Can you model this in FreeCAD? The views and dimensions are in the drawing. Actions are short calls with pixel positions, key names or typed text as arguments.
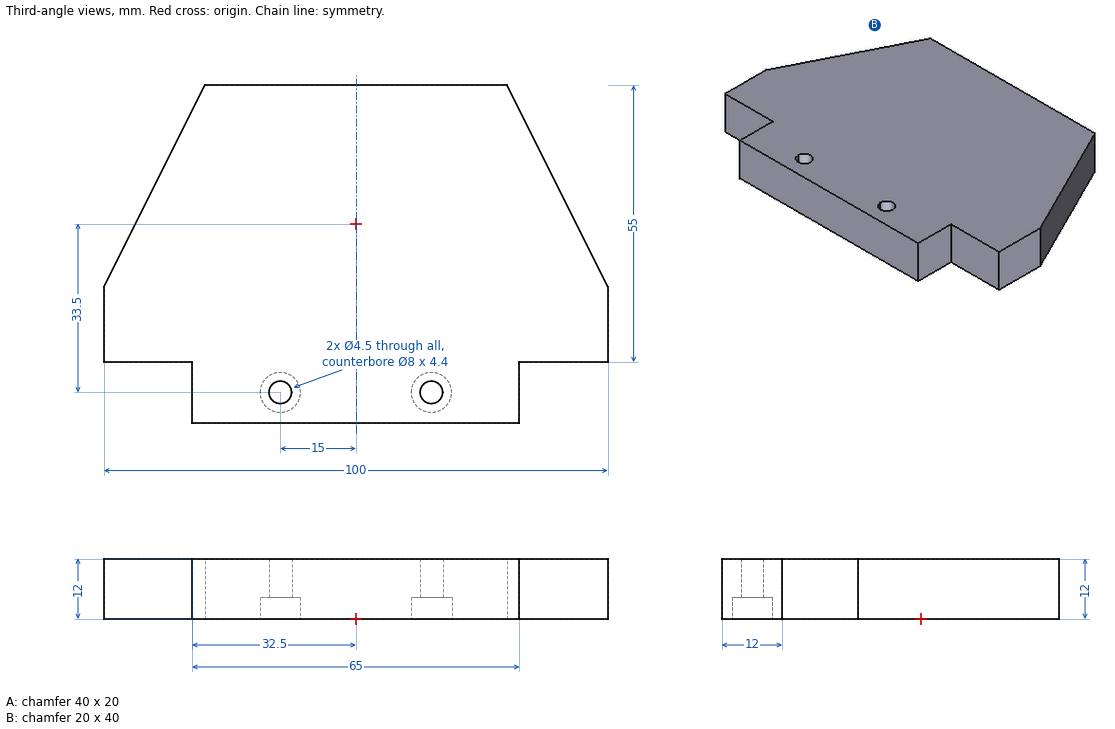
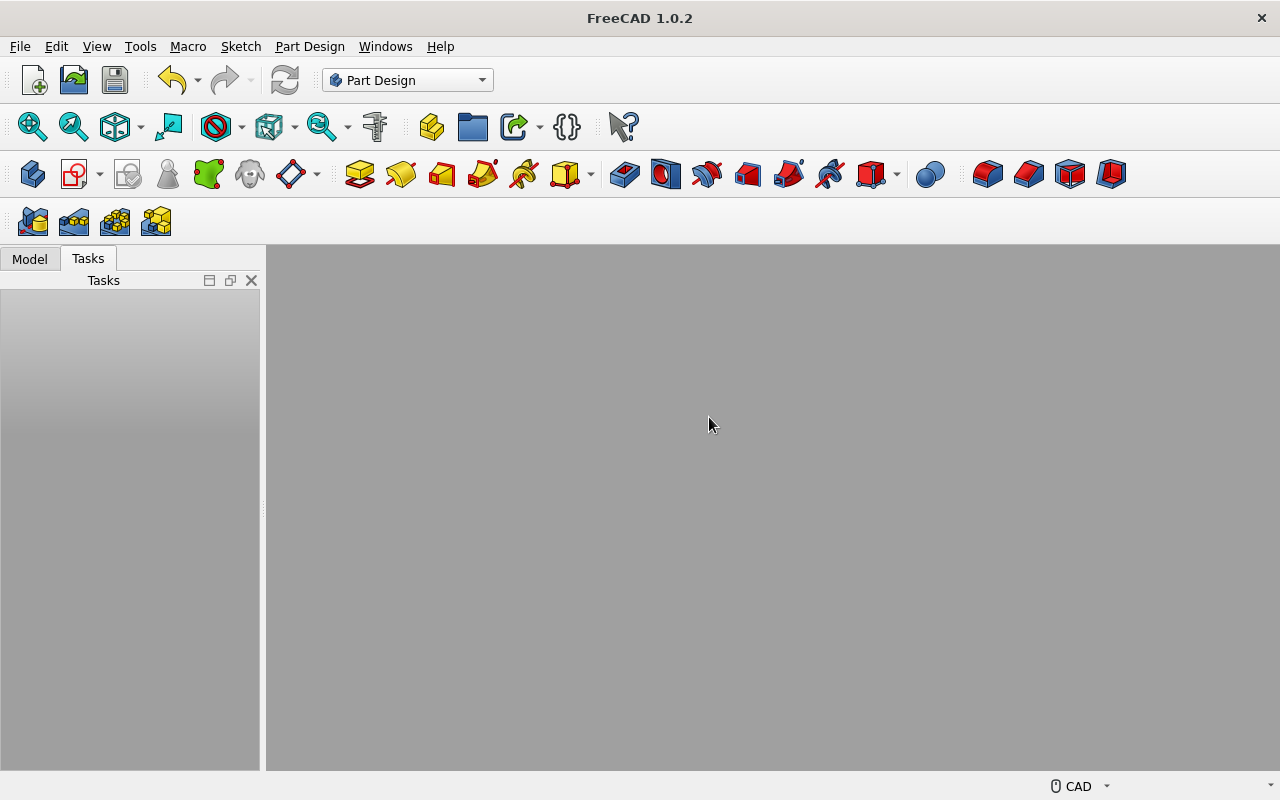
click(33, 80)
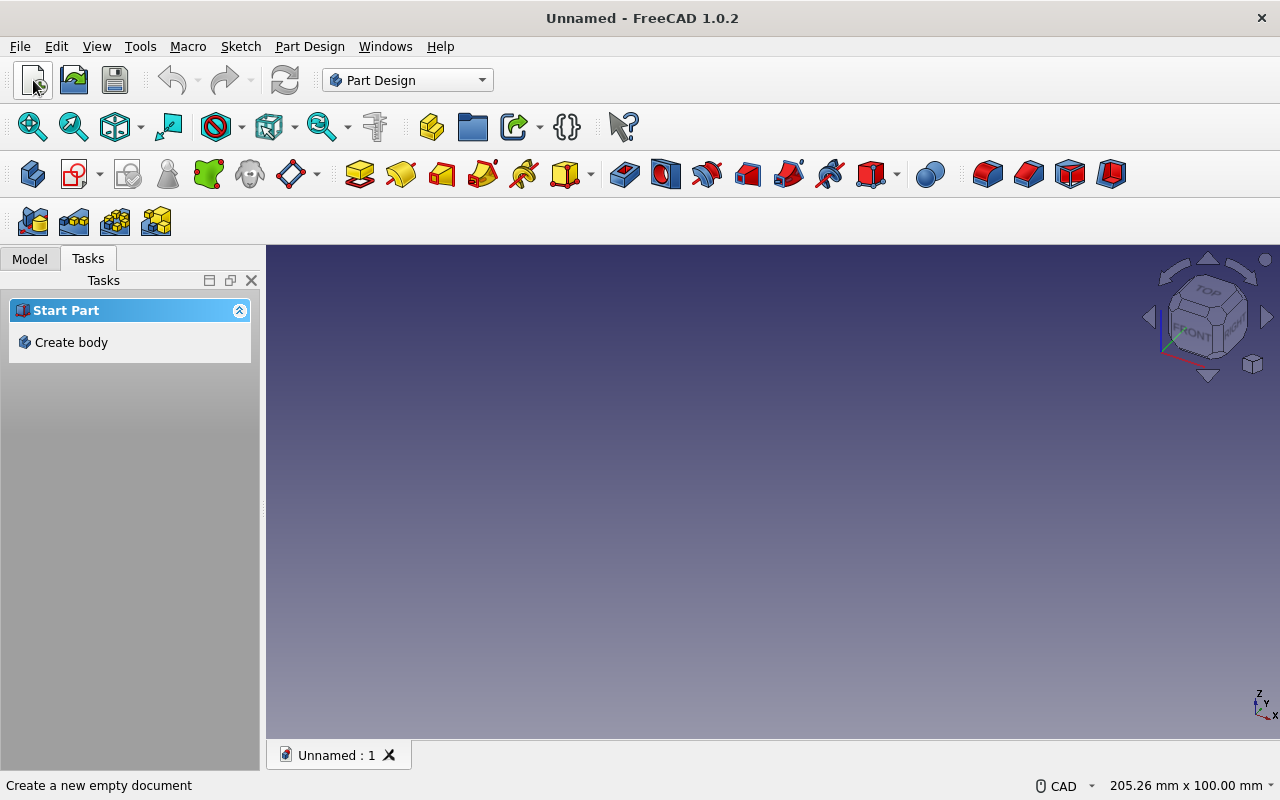
click(74, 174)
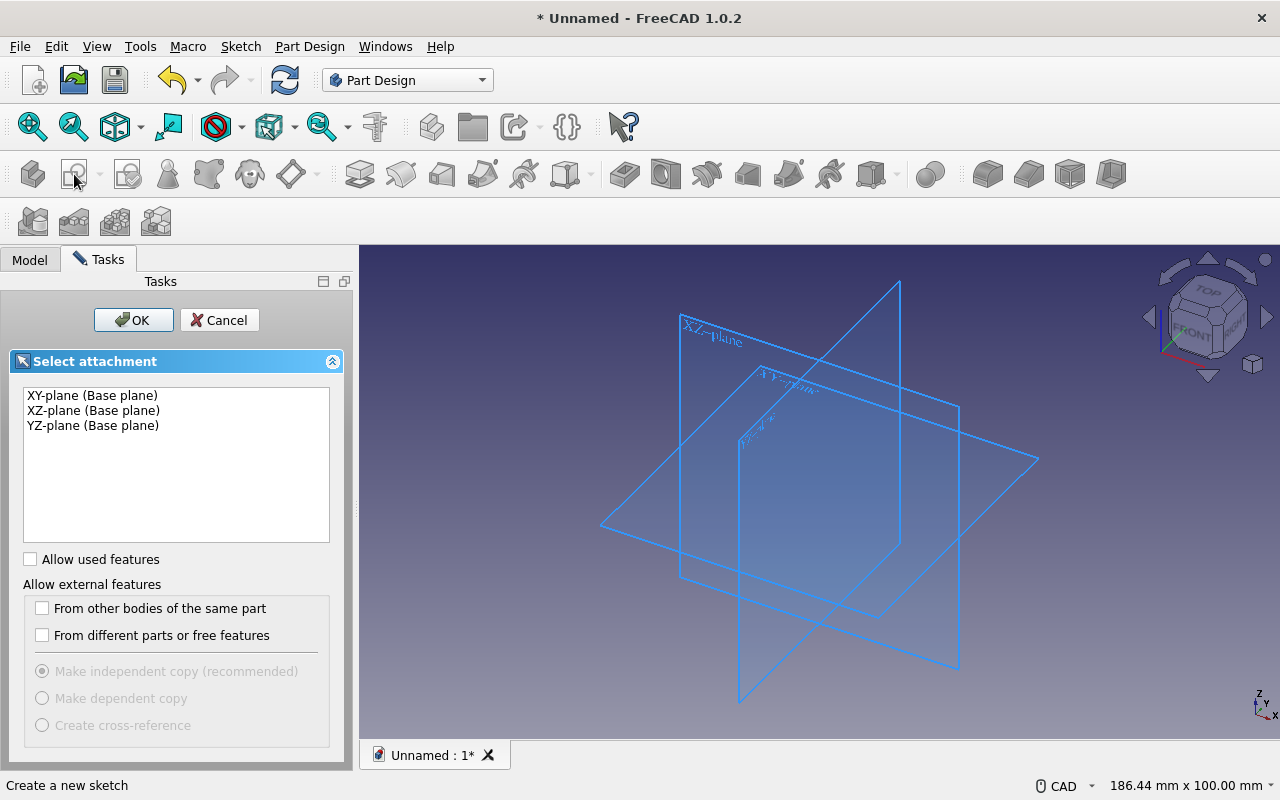
click(84, 396)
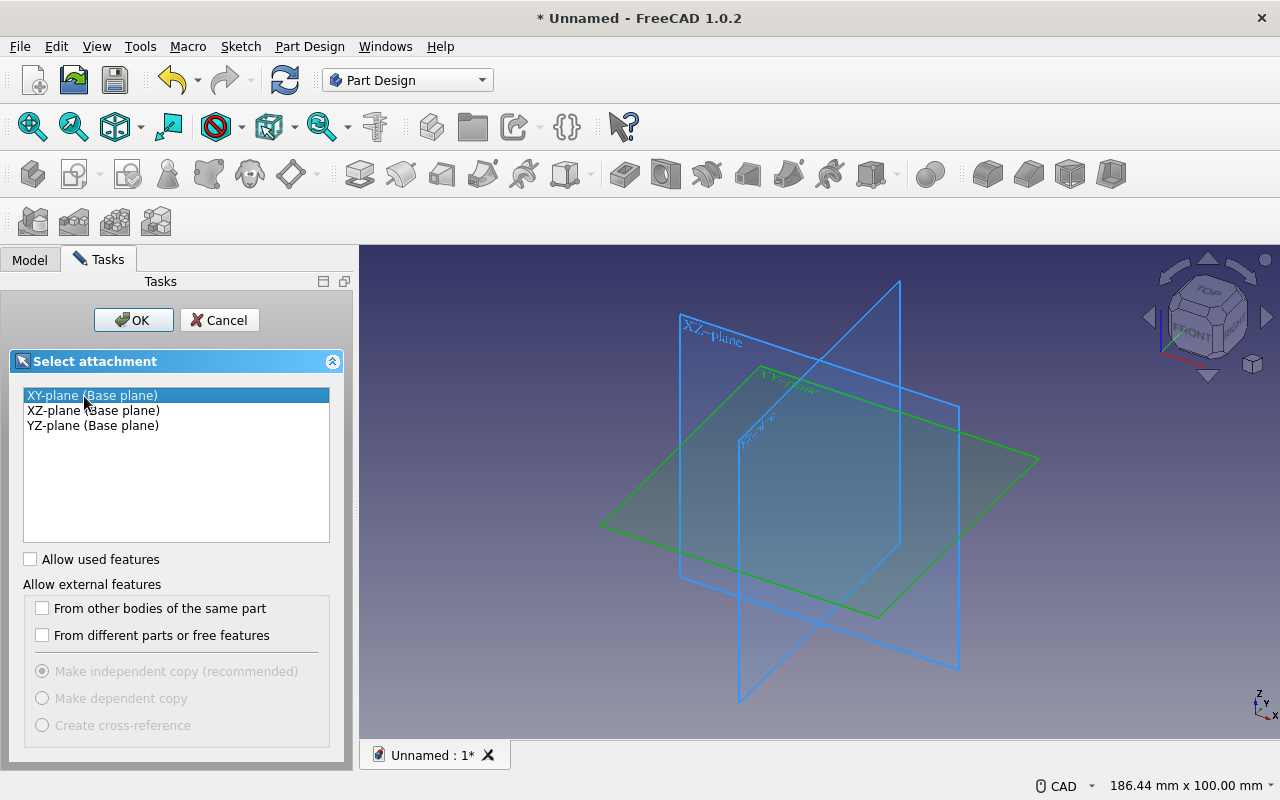
click(134, 320)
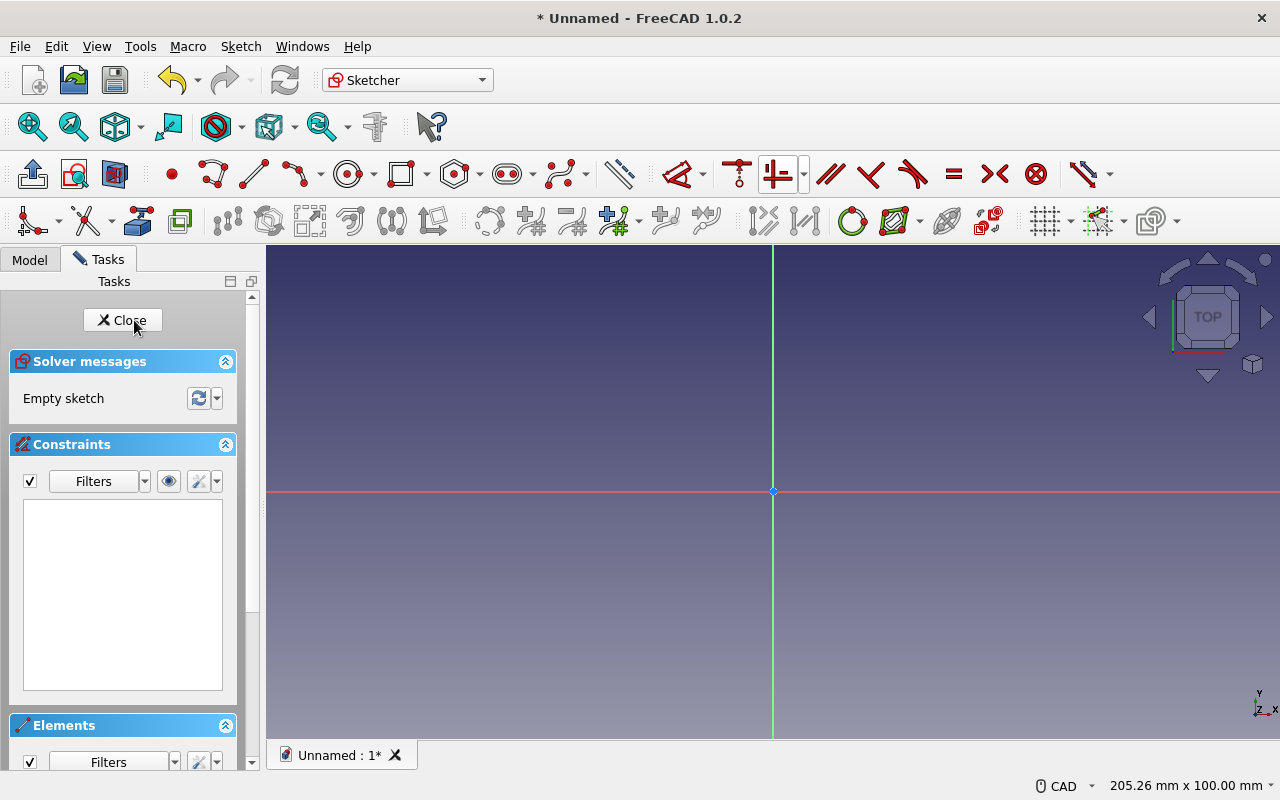
click(426, 174)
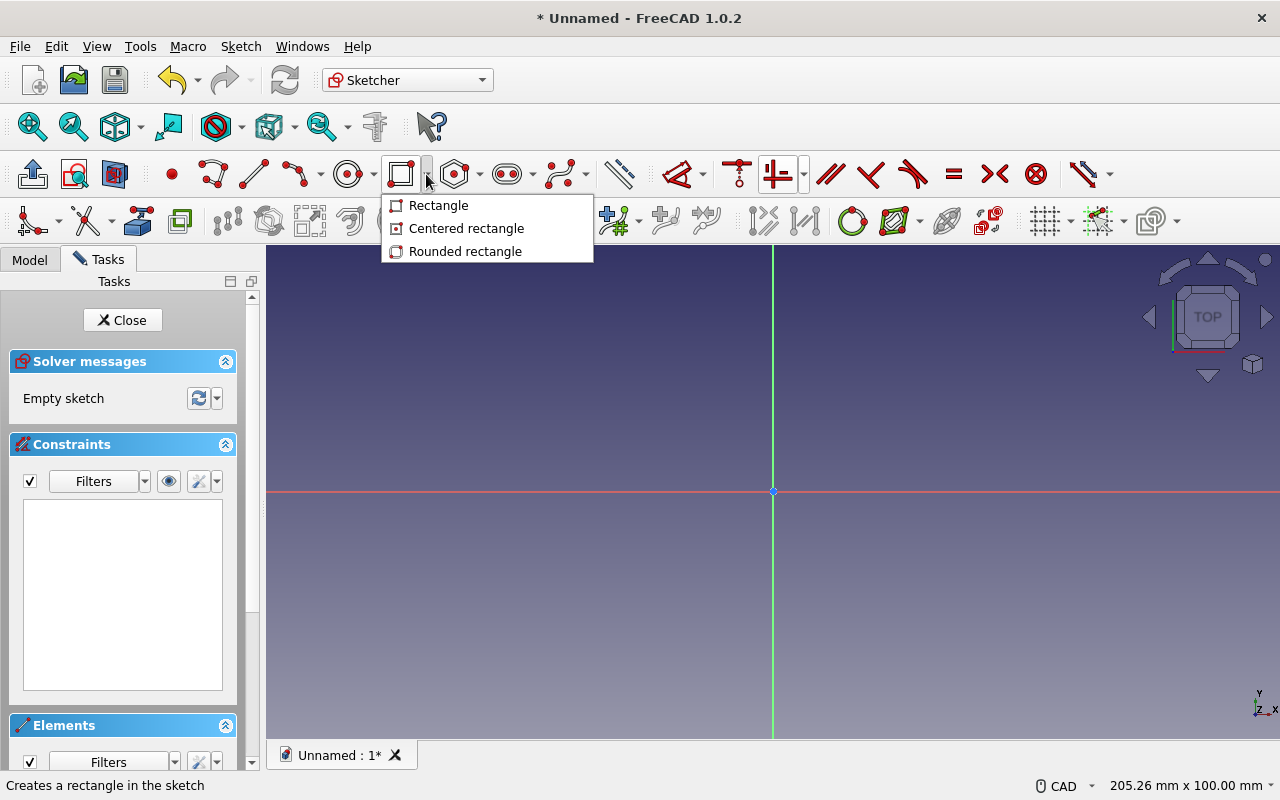
click(488, 228)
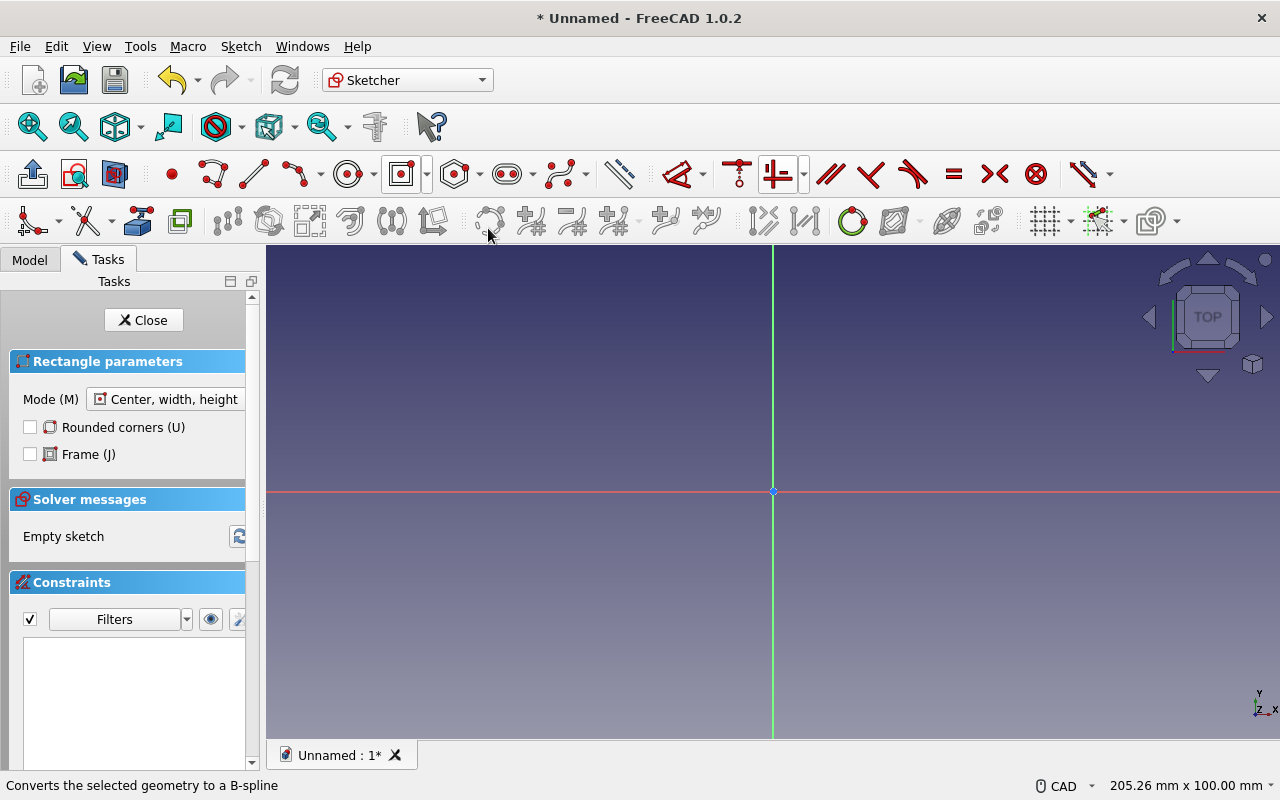
click(773, 492)
move(1020, 356)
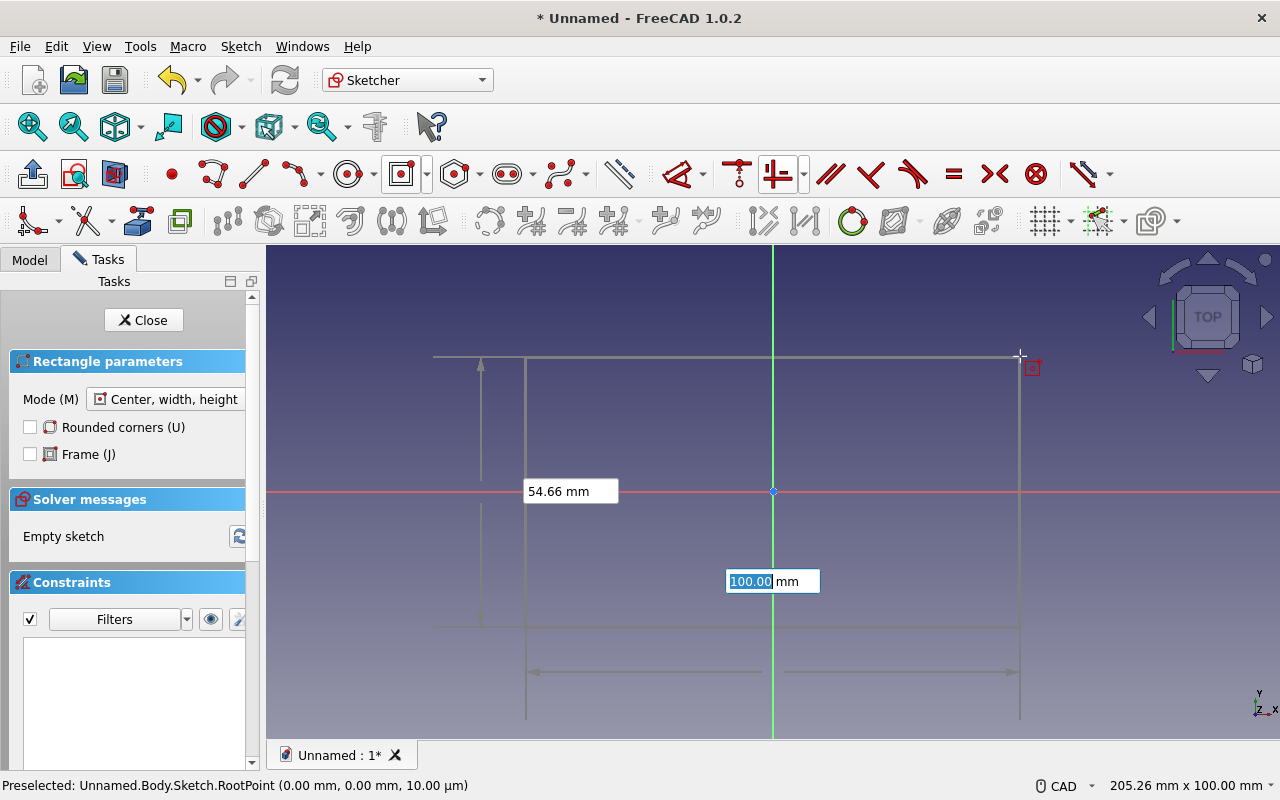
text(100)
key(Tab)
text(55)
key(Return)
key(Escape)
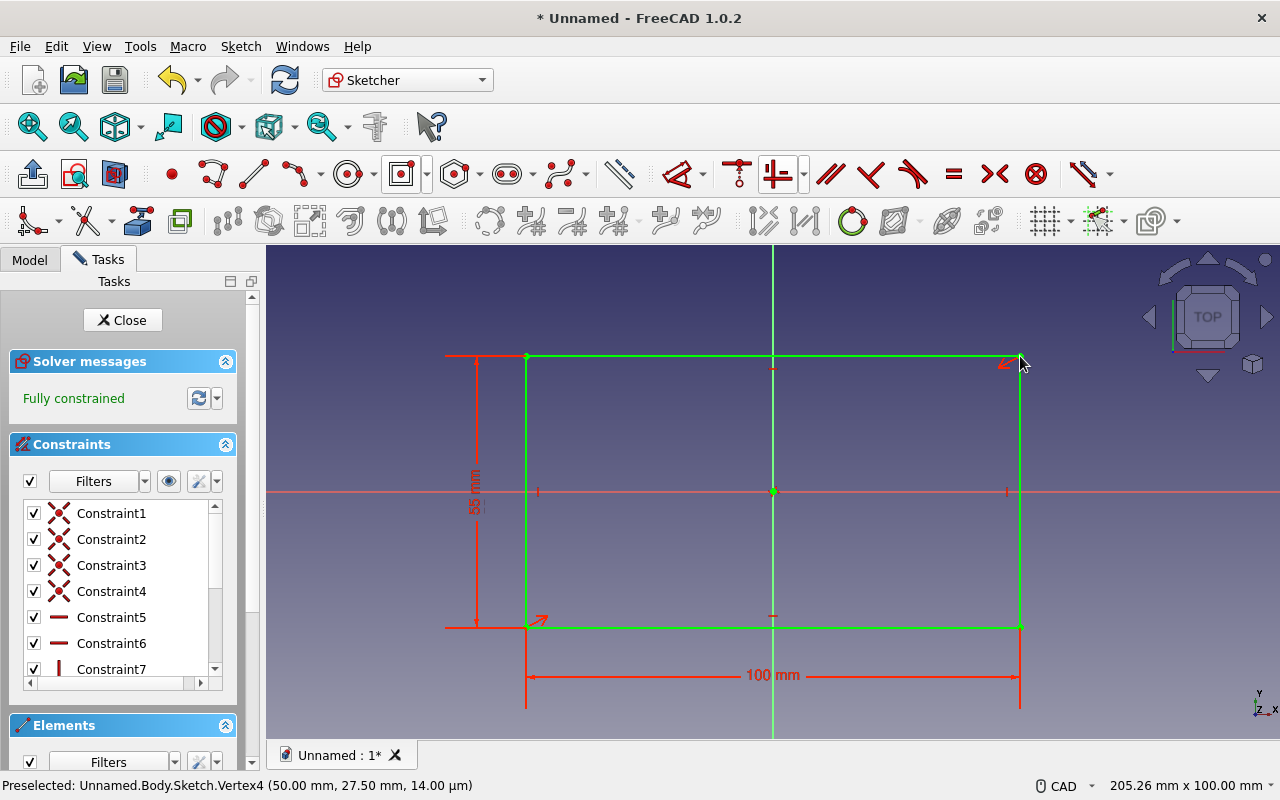
click(123, 320)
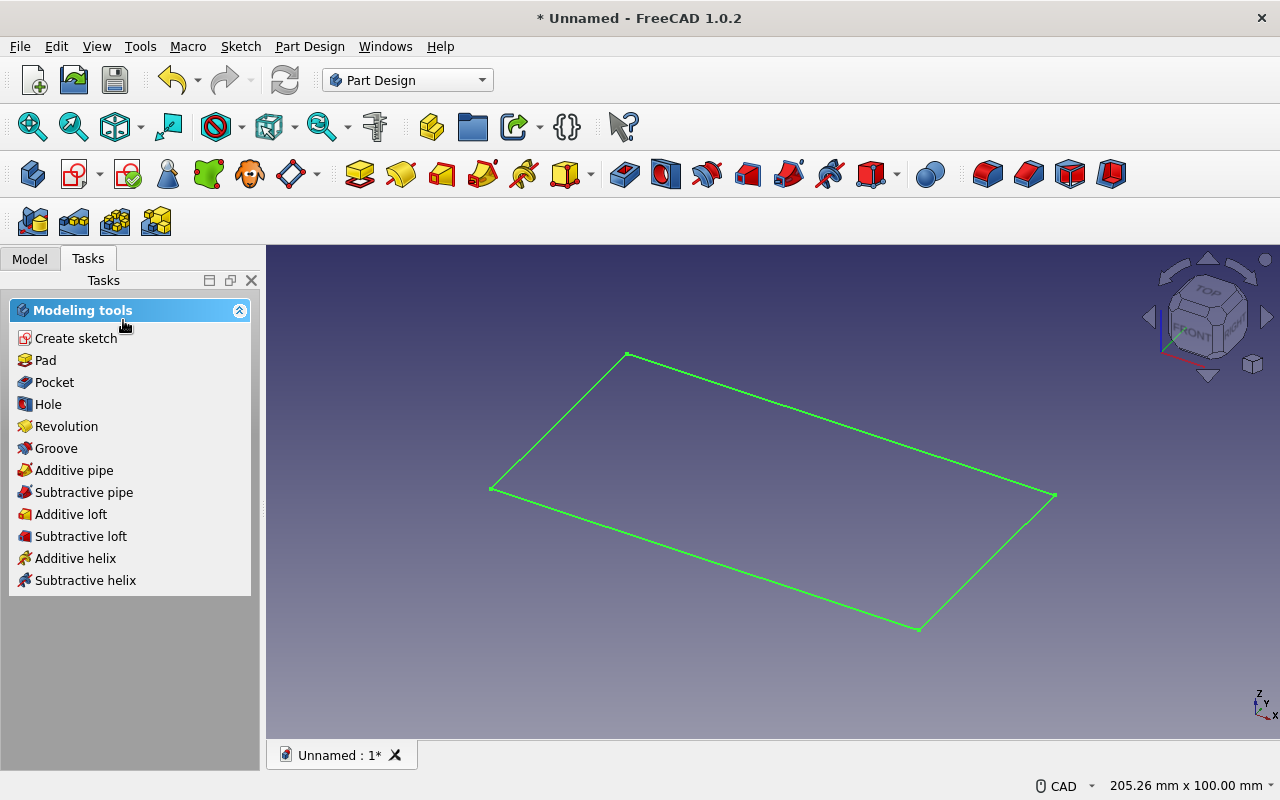
click(360, 174)